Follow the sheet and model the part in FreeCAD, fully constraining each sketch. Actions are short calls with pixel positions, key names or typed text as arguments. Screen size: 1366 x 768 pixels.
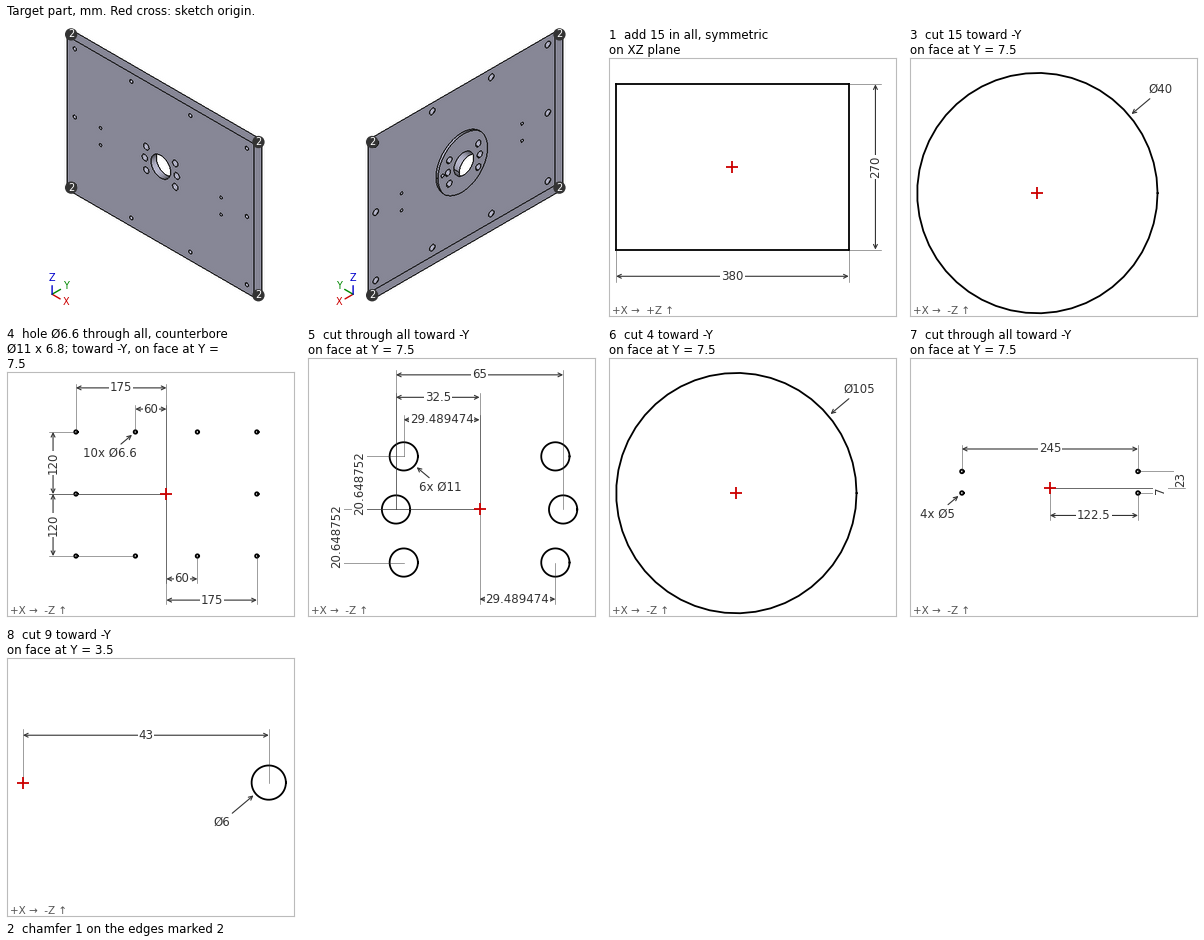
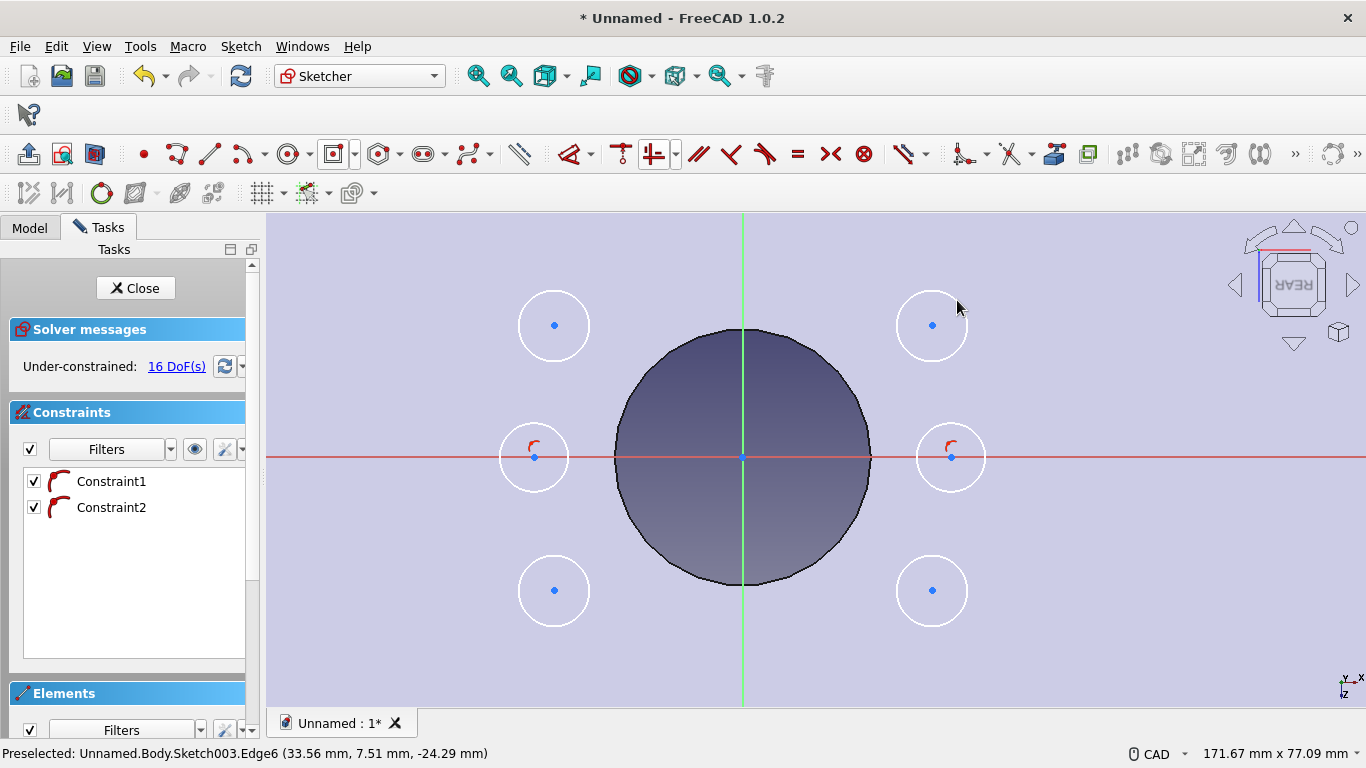
click(579, 301)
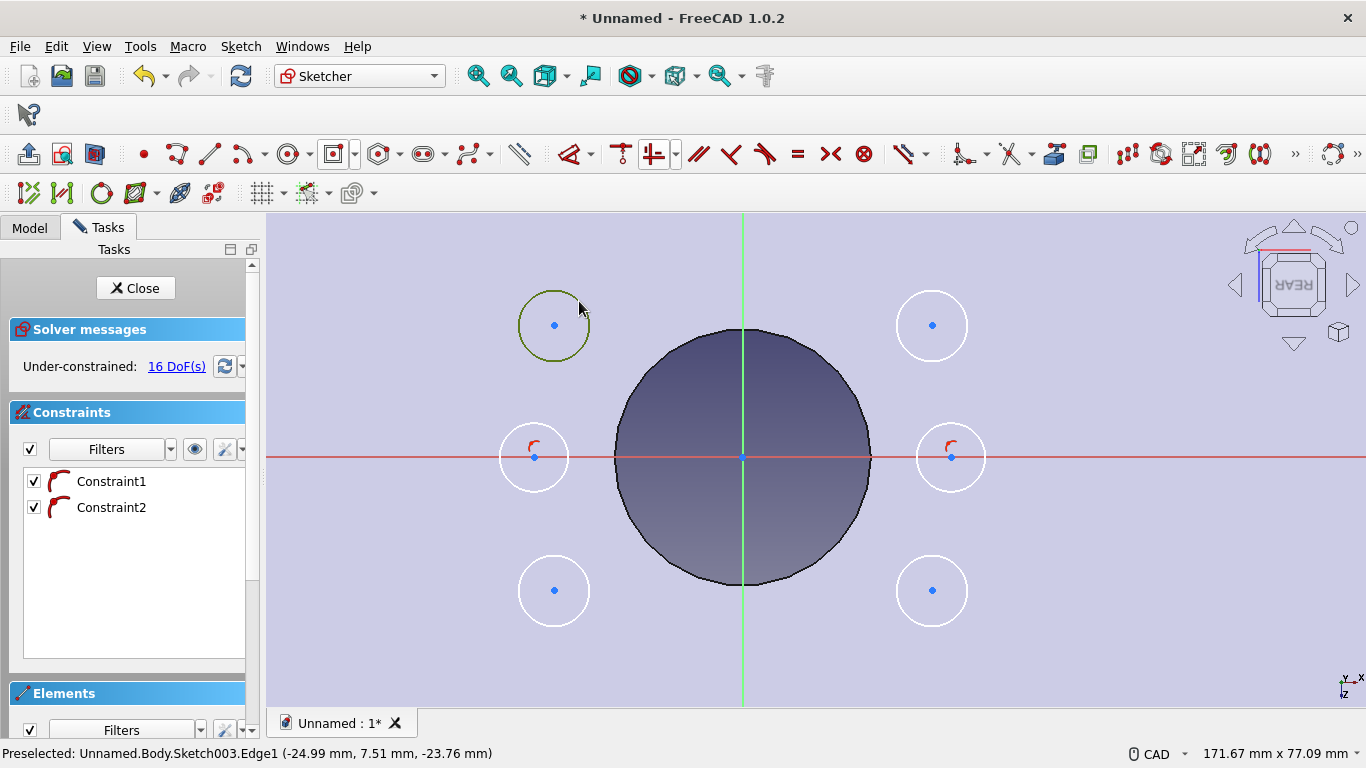
click(579, 566)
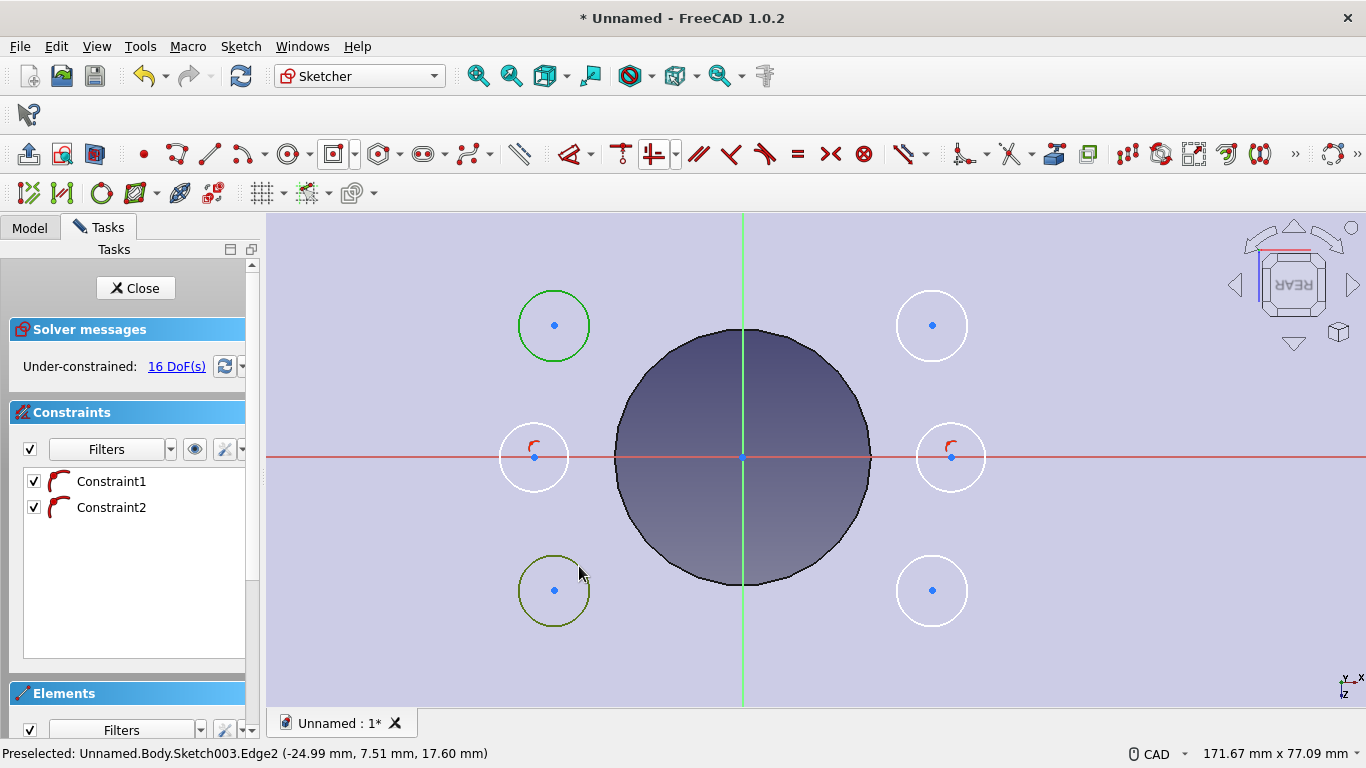
click(558, 433)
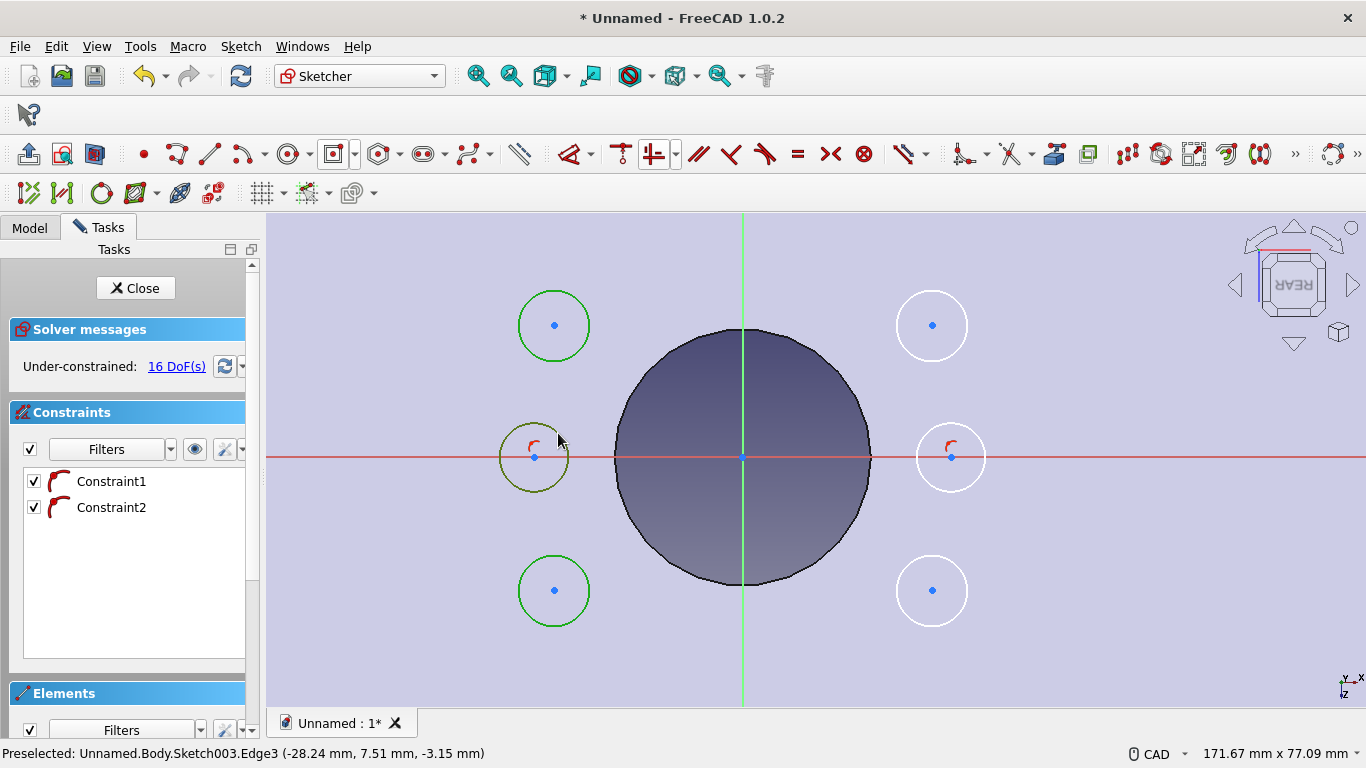
click(957, 566)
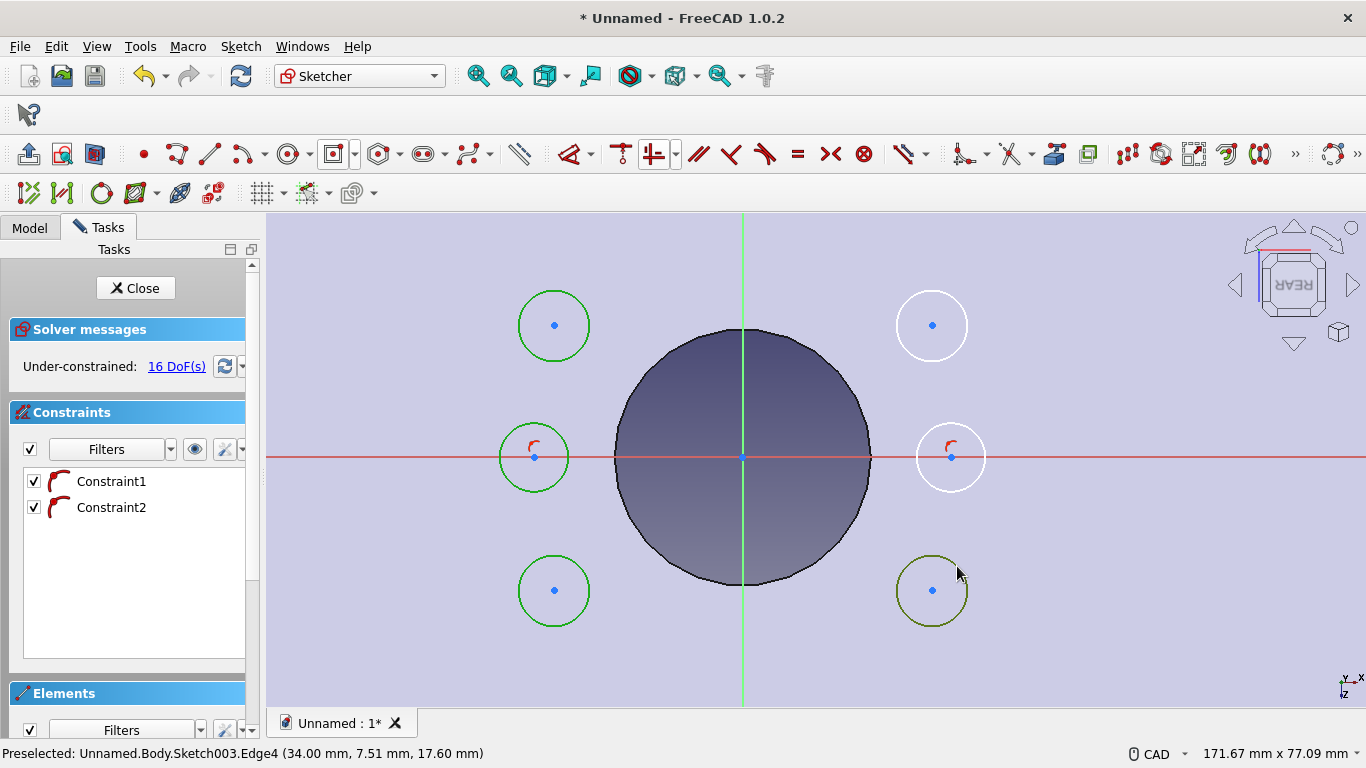
click(975, 433)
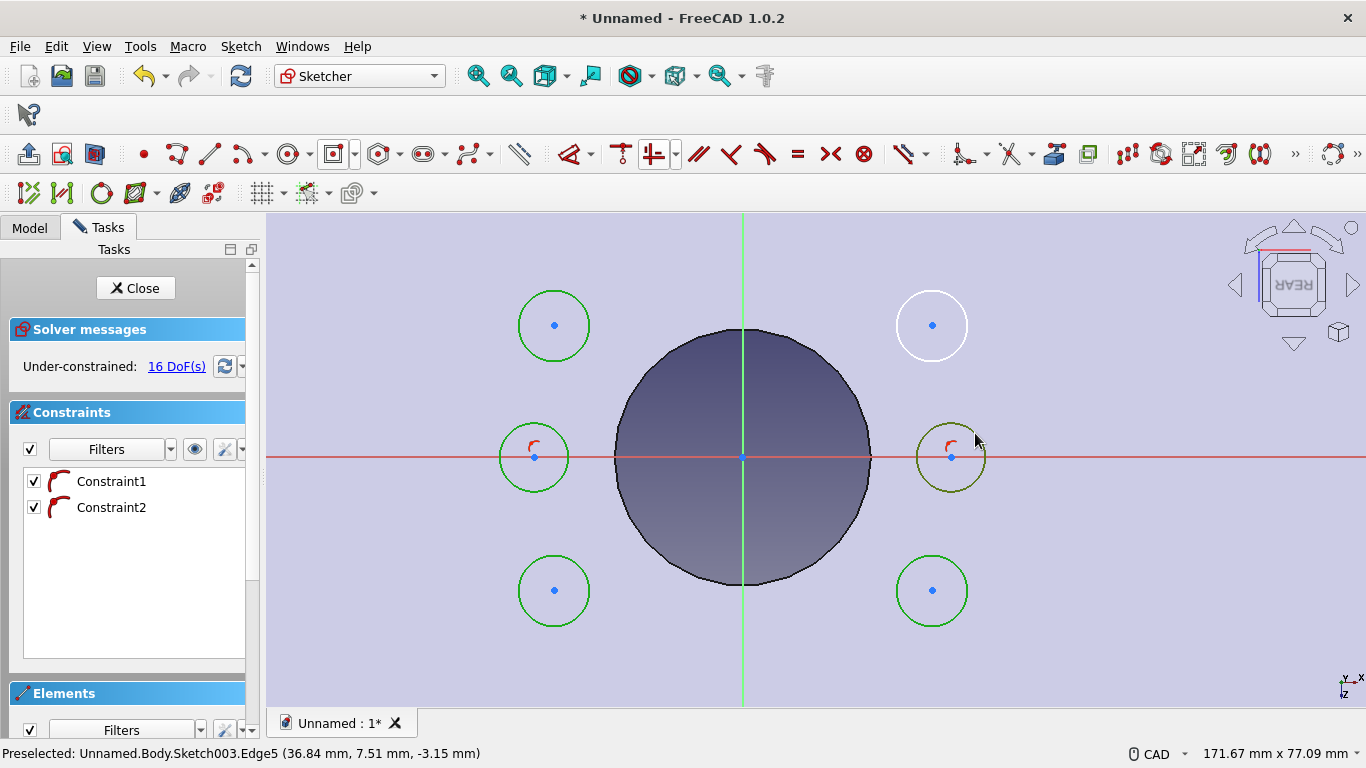
click(957, 301)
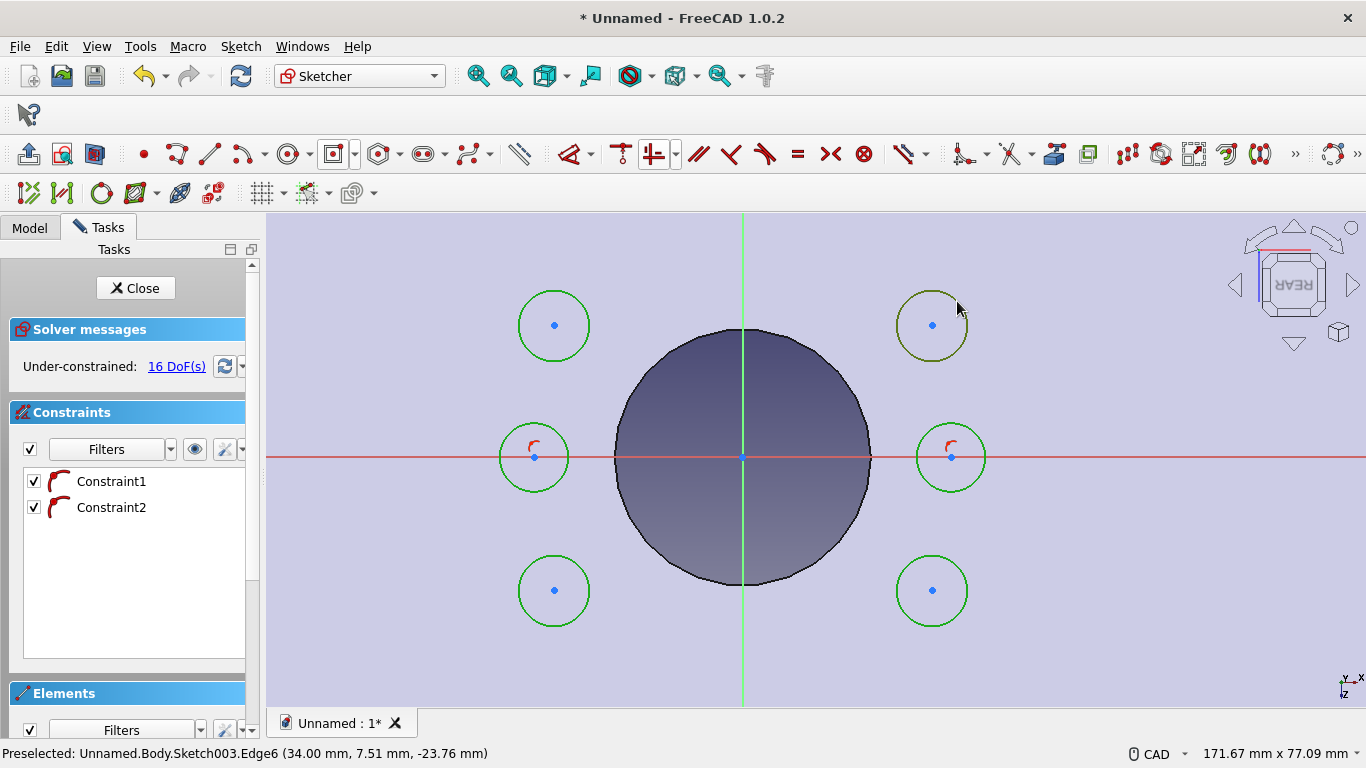
click(798, 154)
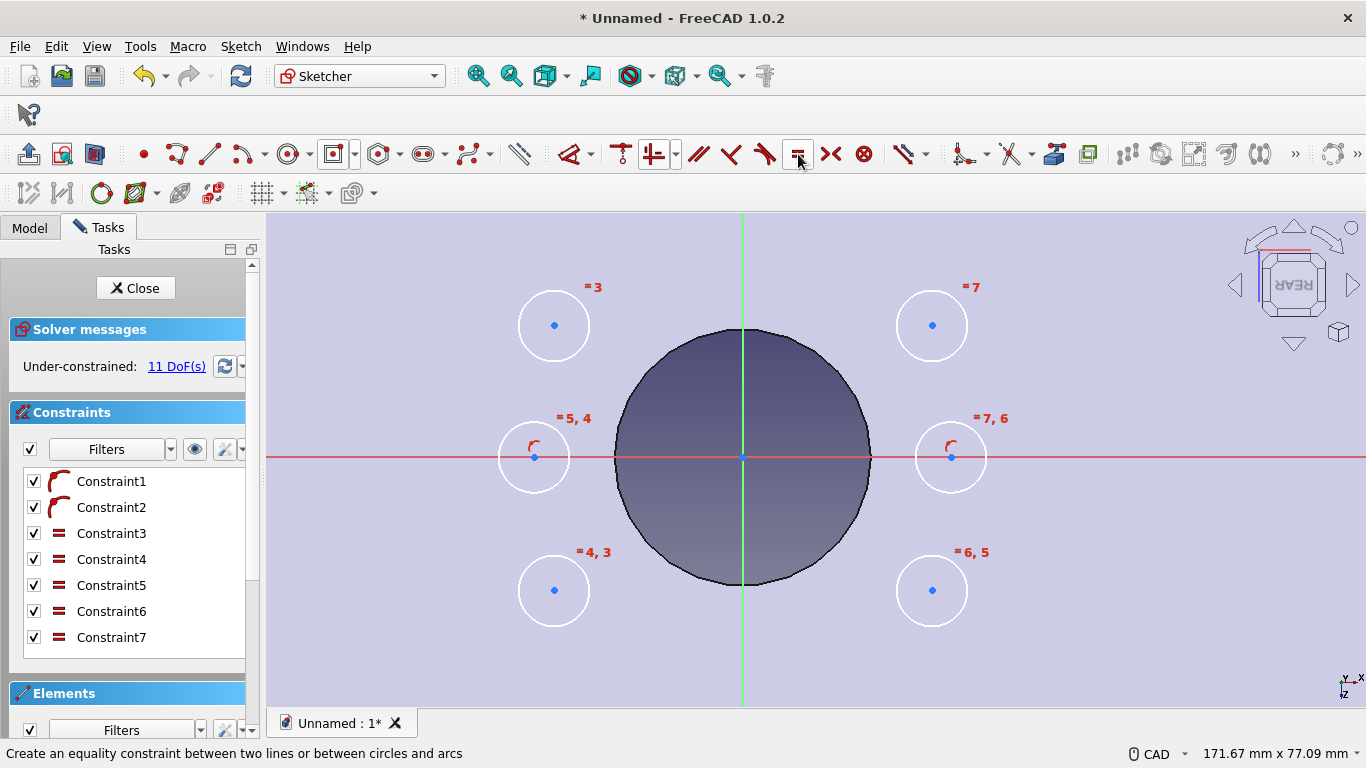
click(554, 326)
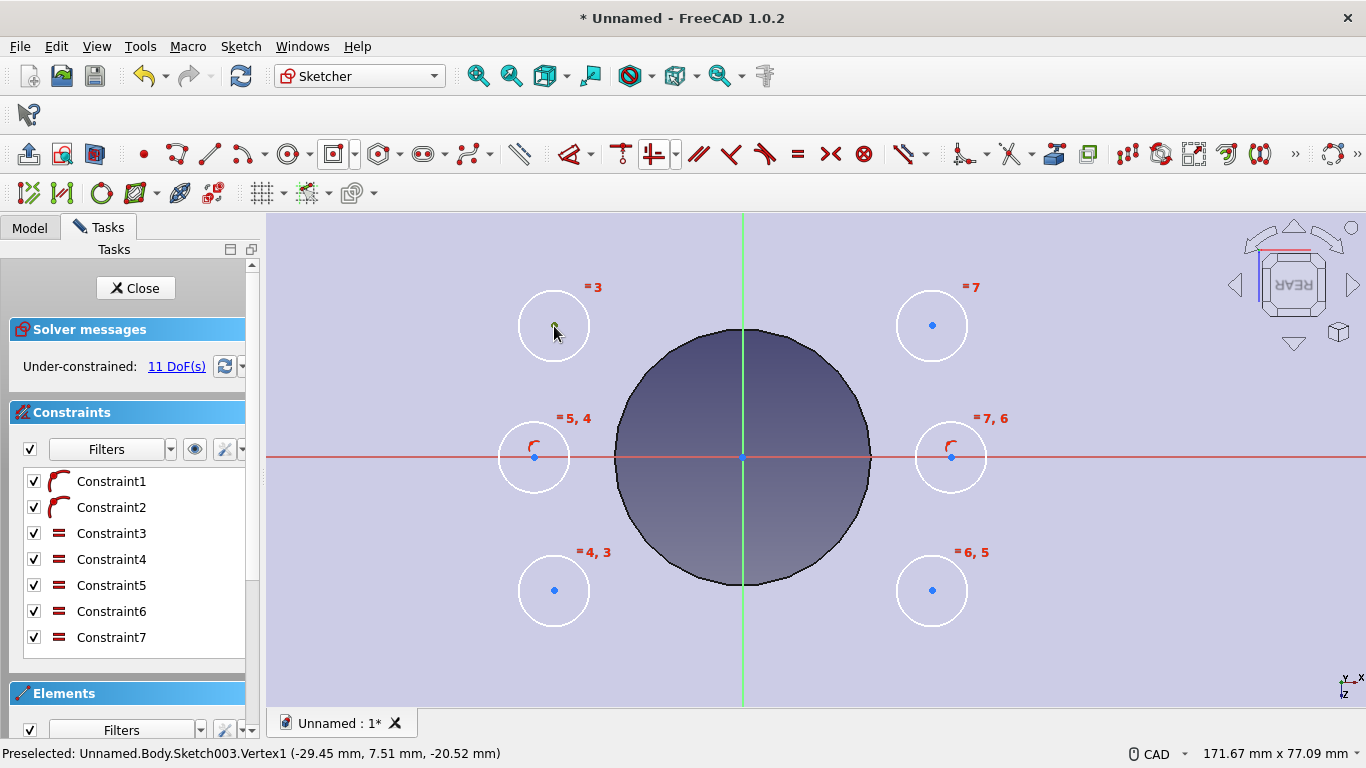
click(554, 591)